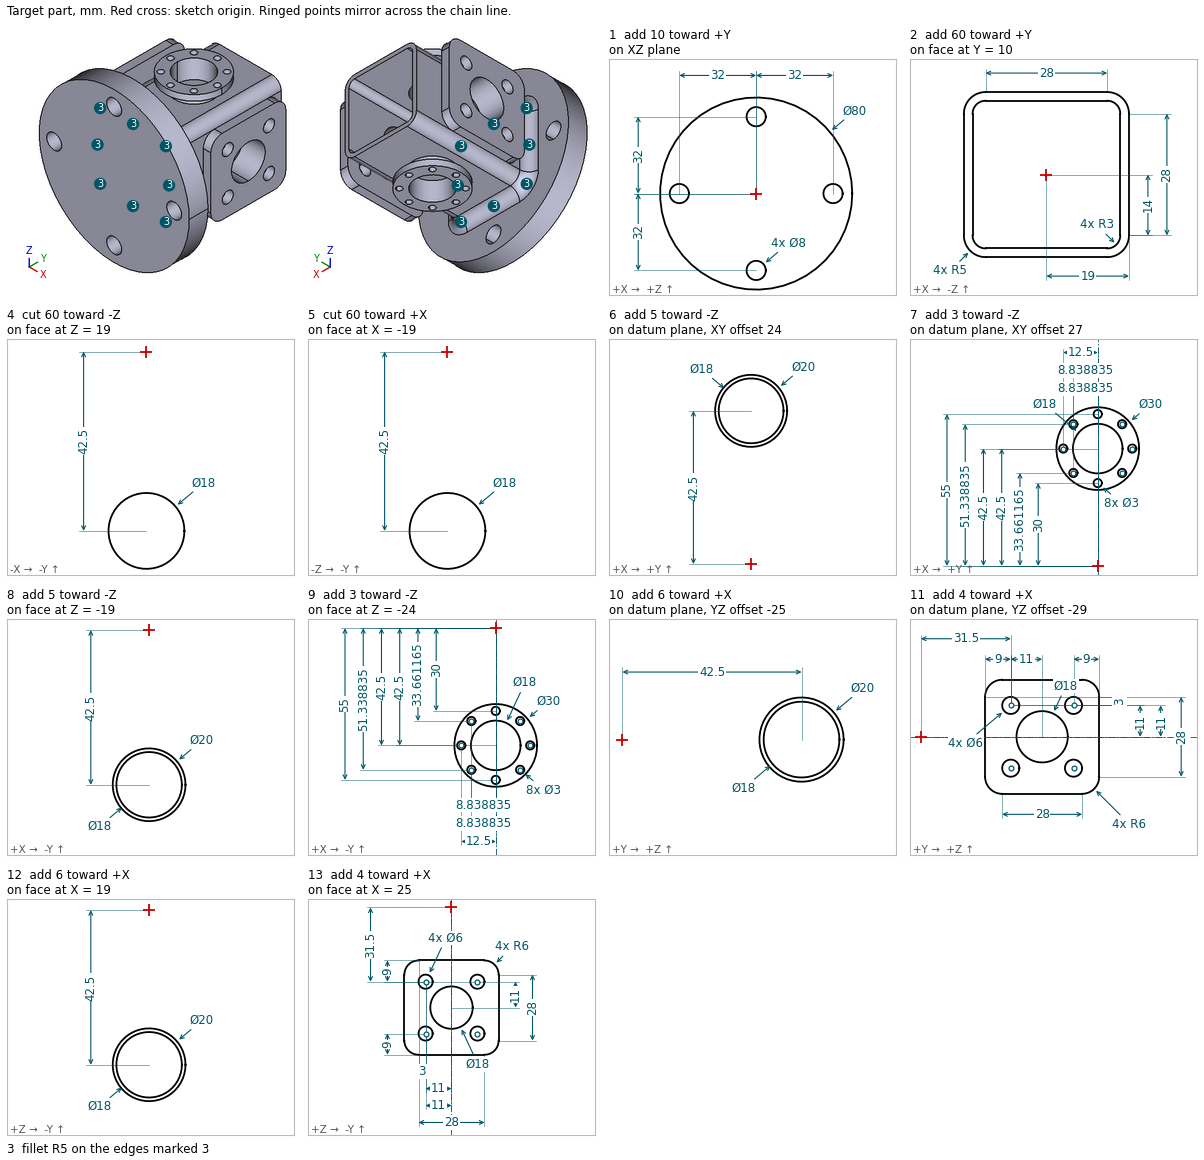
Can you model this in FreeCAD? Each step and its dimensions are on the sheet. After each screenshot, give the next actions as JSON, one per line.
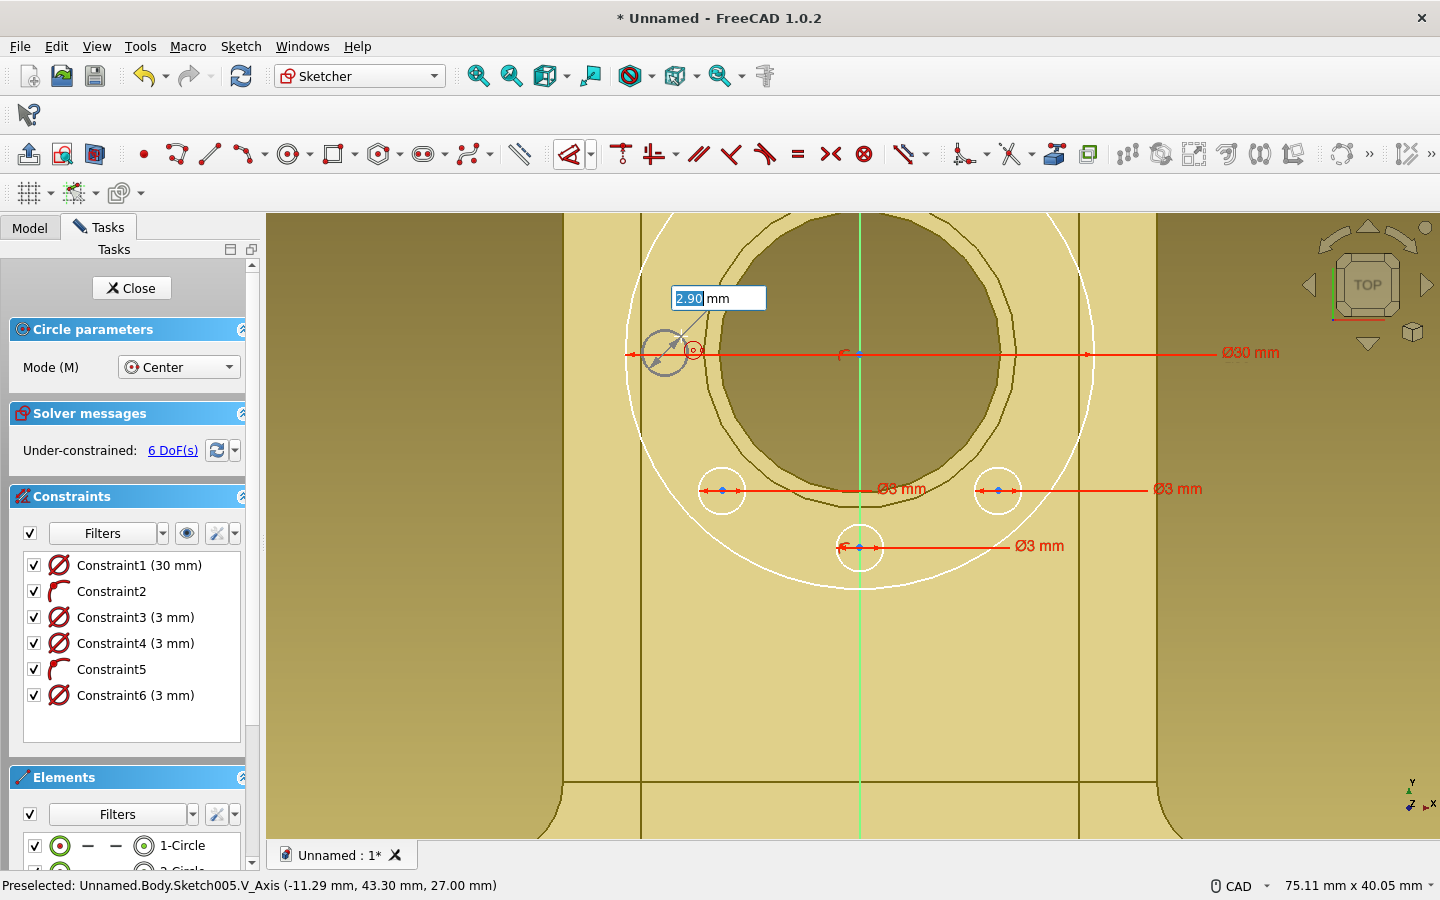
{"action": "type", "text": "3"}
{"action": "key", "text": "Return"}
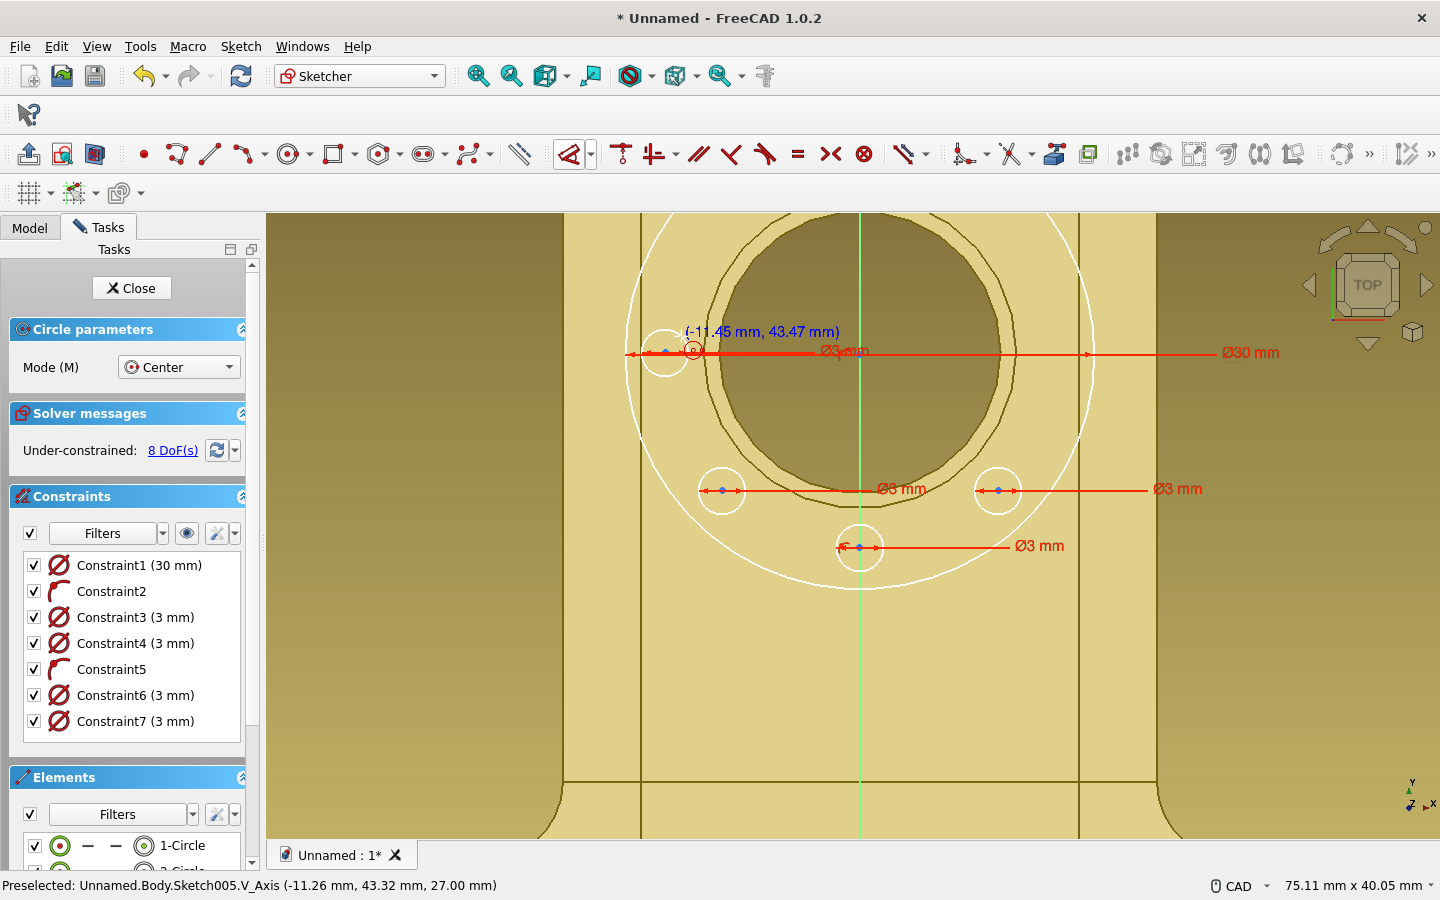
{"action": "scroll", "coordinate": [723, 493], "scroll_direction": "down", "scroll_amount": 4}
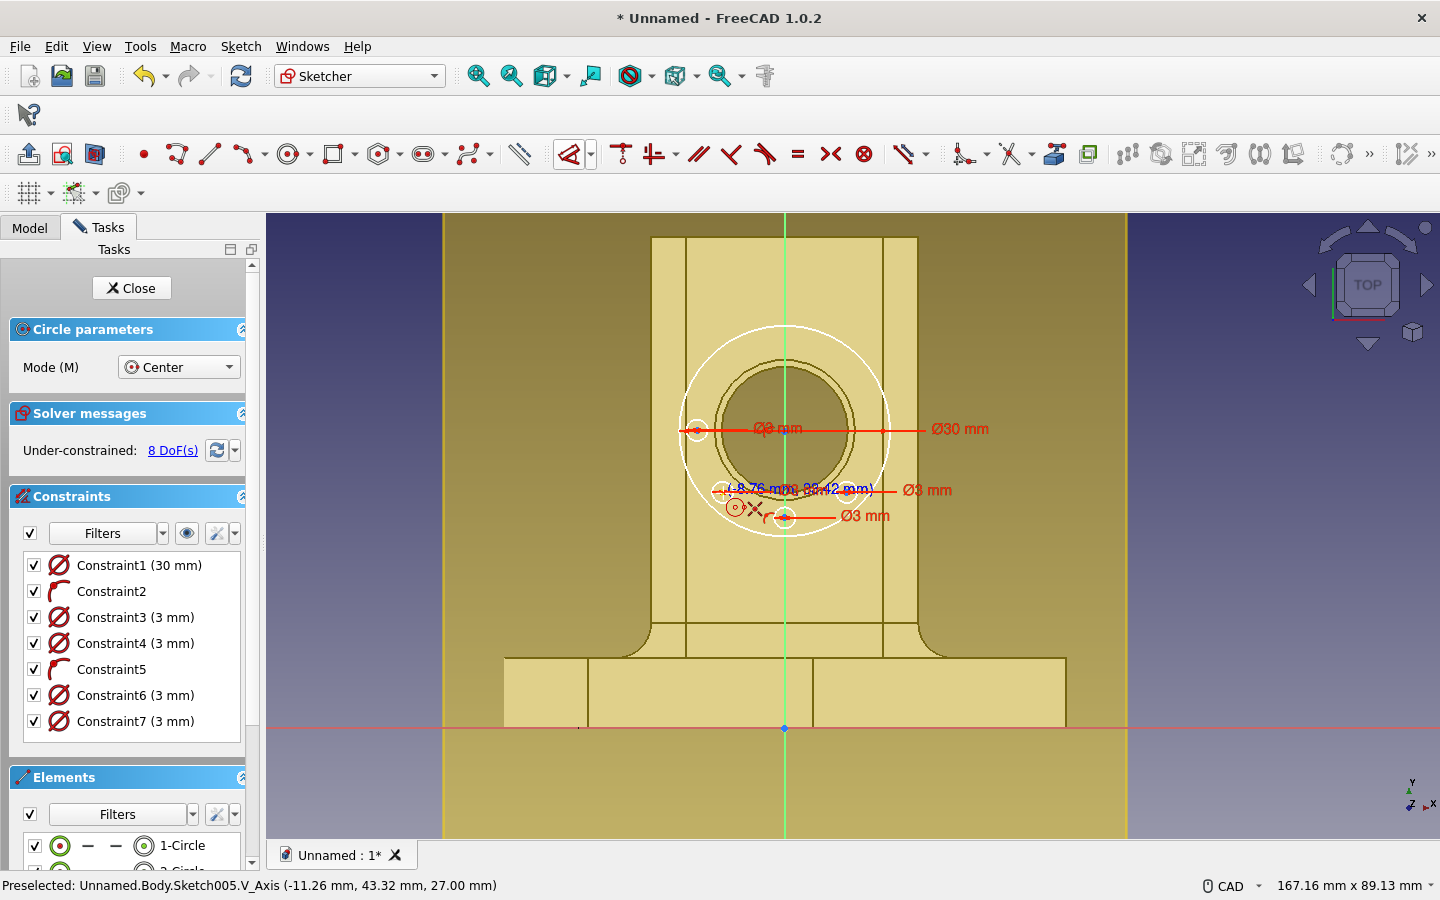
{"action": "scroll", "coordinate": [723, 368], "scroll_direction": "up", "scroll_amount": 4}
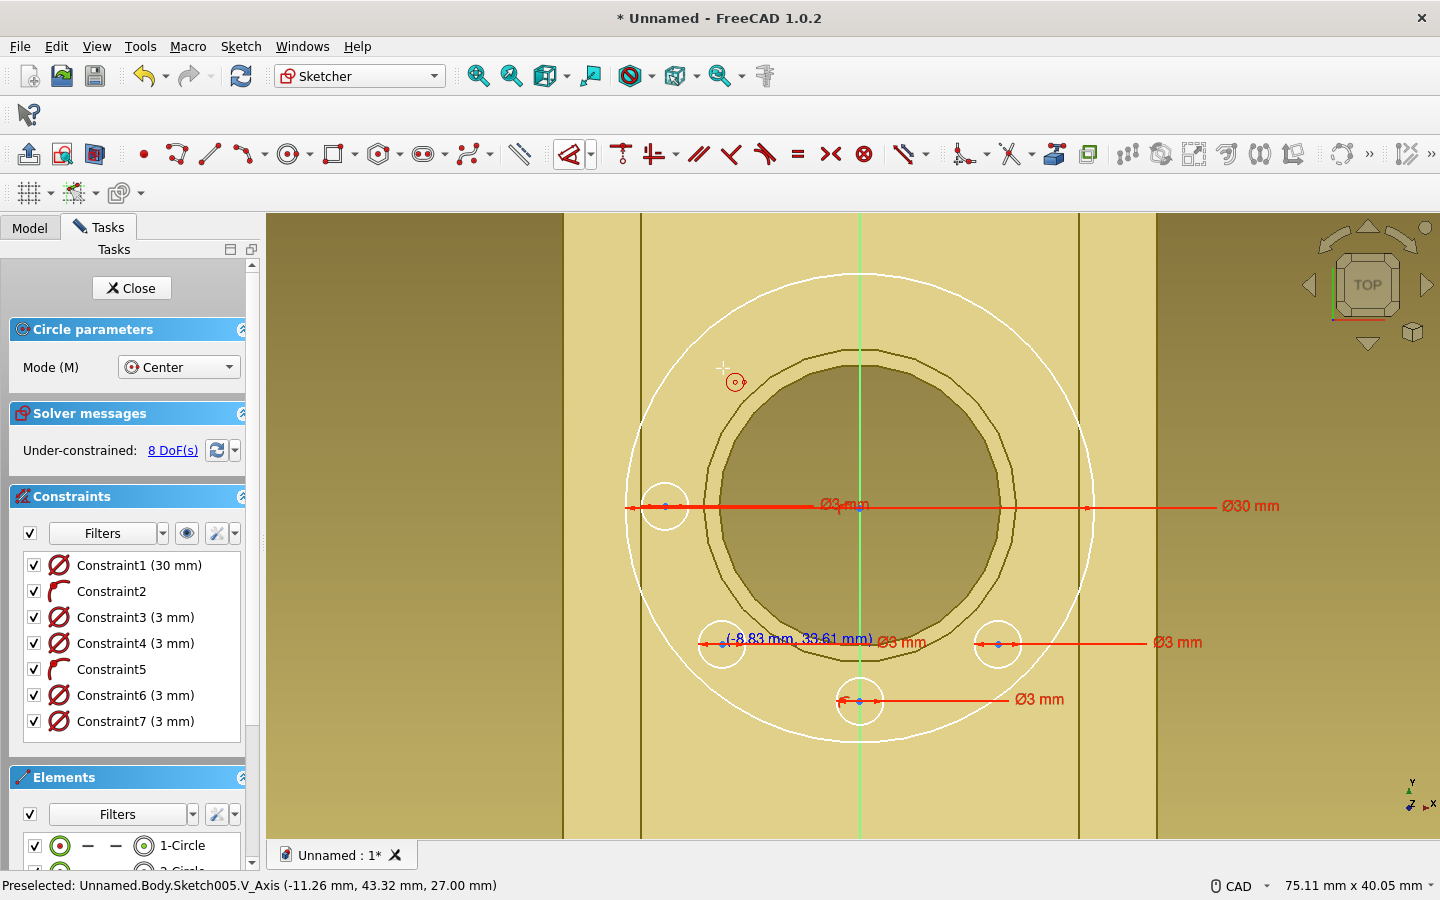
{"action": "left_click", "coordinate": [722, 367]}
{"action": "mouse_move", "coordinate": [738, 351]}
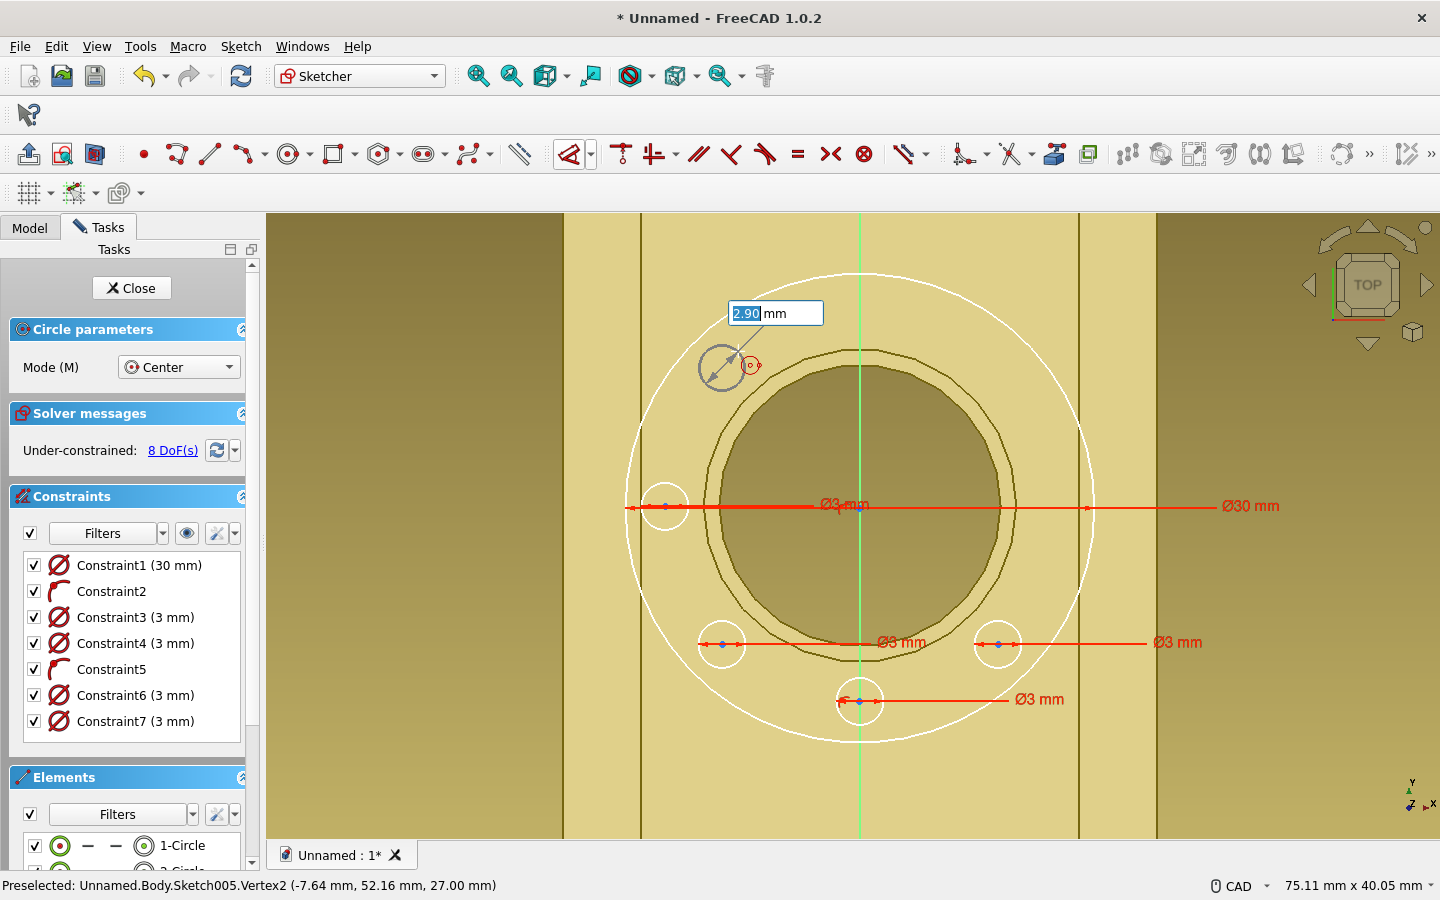
{"action": "type", "text": "3"}
{"action": "key", "text": "Return"}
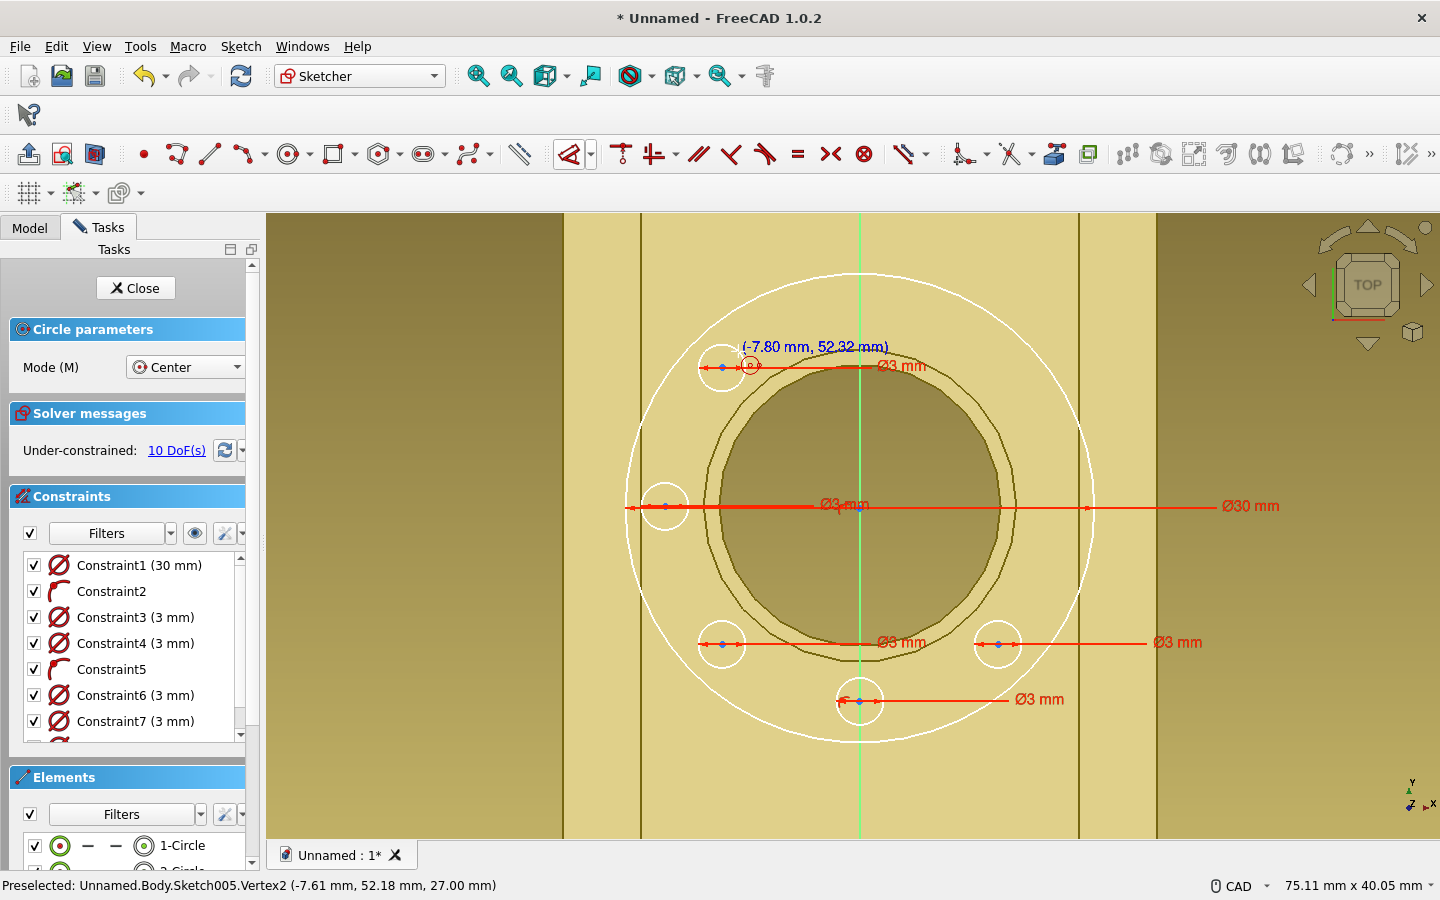
{"action": "left_click", "coordinate": [860, 508]}
{"action": "mouse_move", "coordinate": [959, 406]}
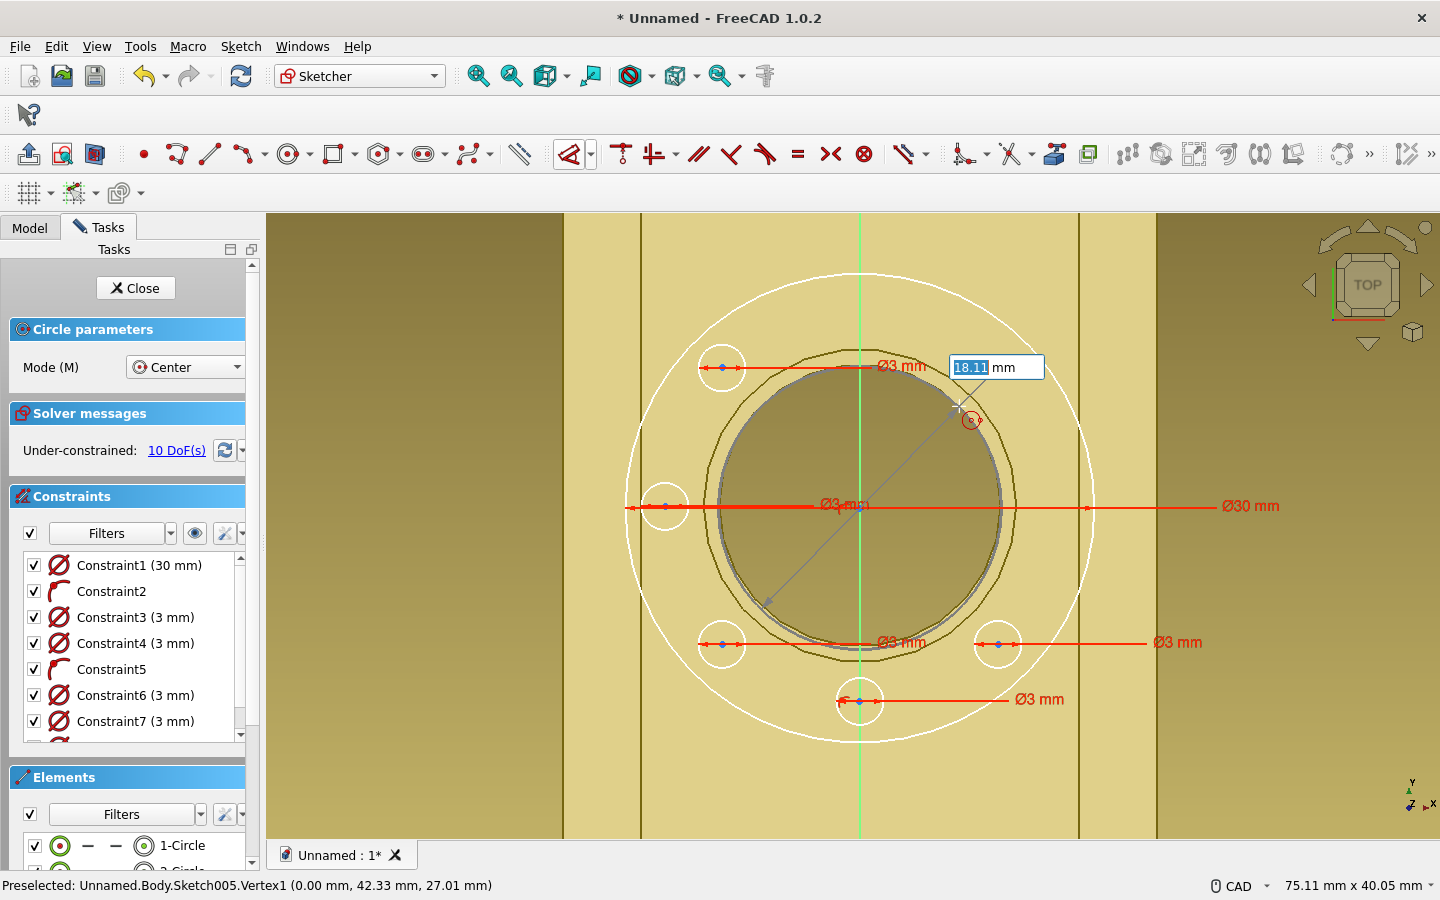
{"action": "type", "text": "18"}
{"action": "key", "text": "Return"}